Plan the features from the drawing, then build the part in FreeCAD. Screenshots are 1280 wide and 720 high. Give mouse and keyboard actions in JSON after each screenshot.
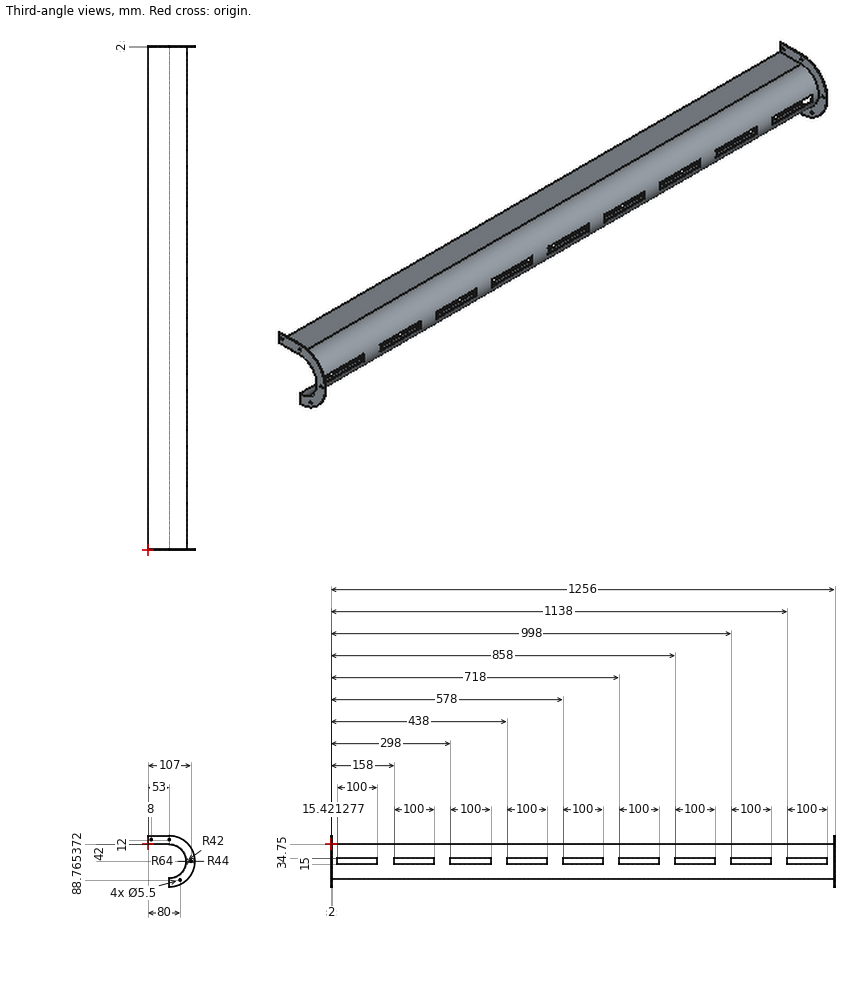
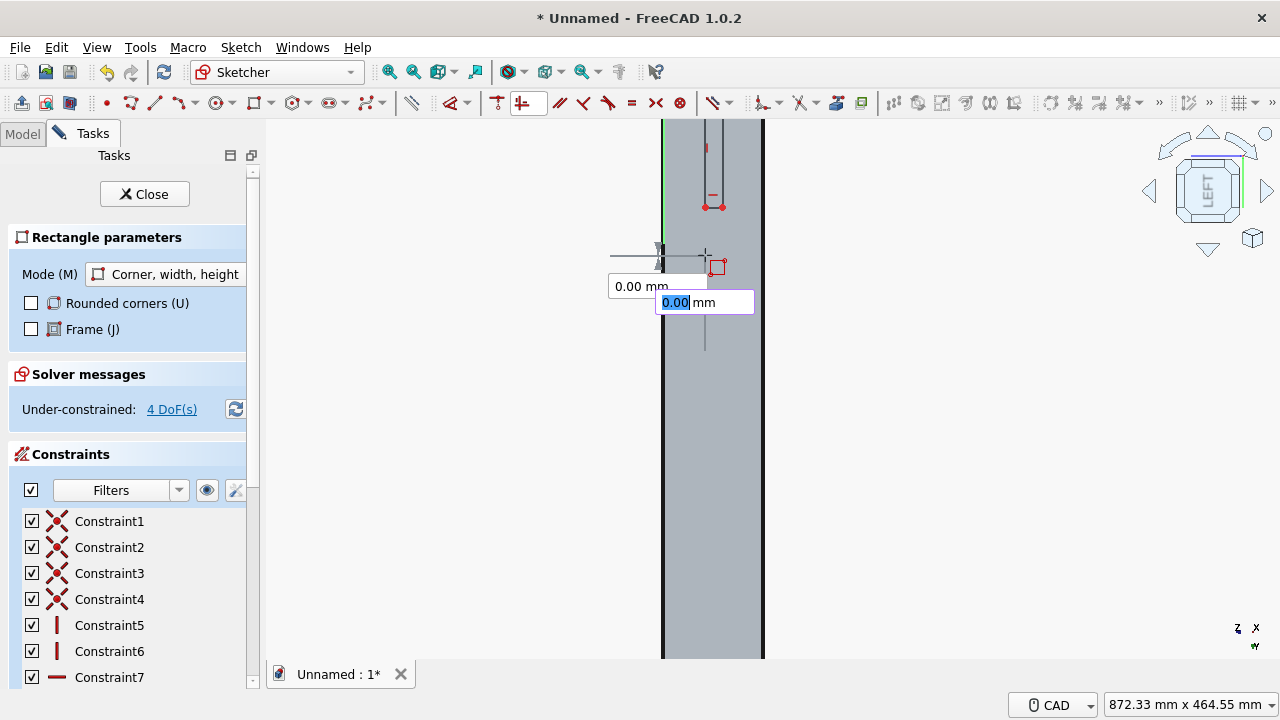
{"action": "scroll", "coordinate": [708, 258], "scroll_direction": "down", "scroll_amount": 7}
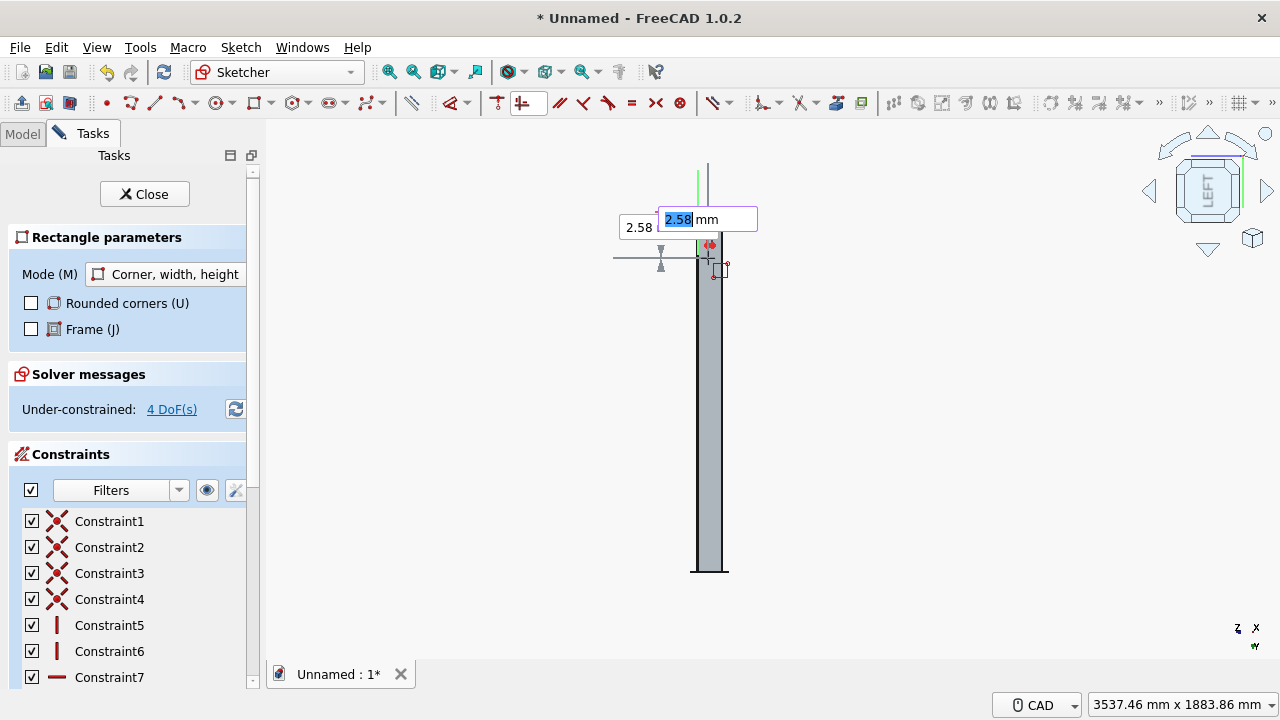
{"action": "left_click", "coordinate": [712, 286]}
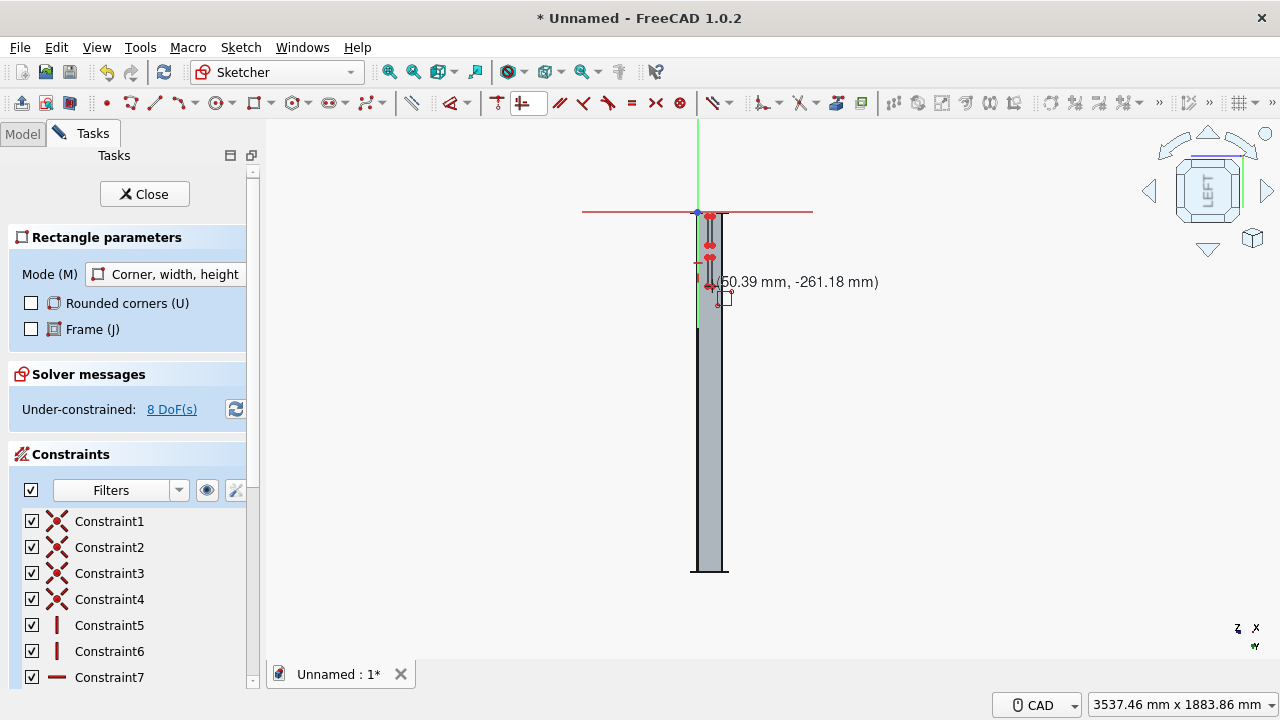
{"action": "scroll", "coordinate": [708, 498], "scroll_direction": "up", "scroll_amount": 7}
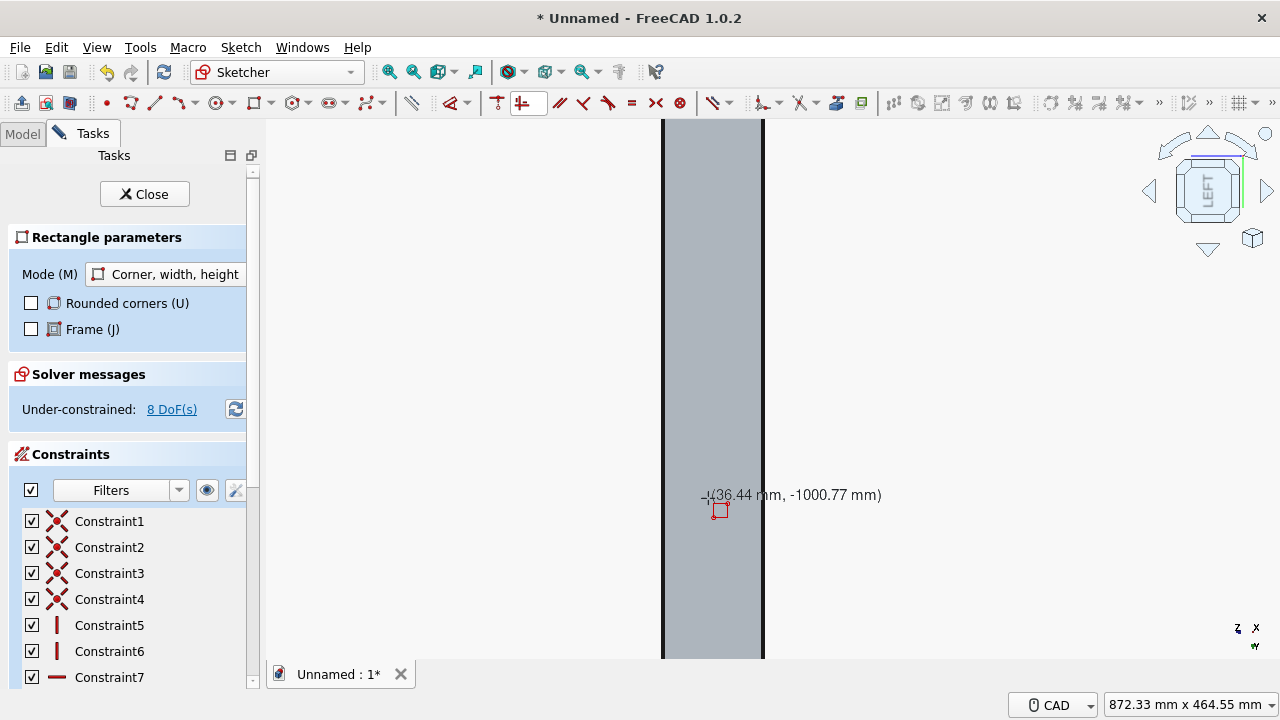
{"action": "left_click", "coordinate": [705, 497]}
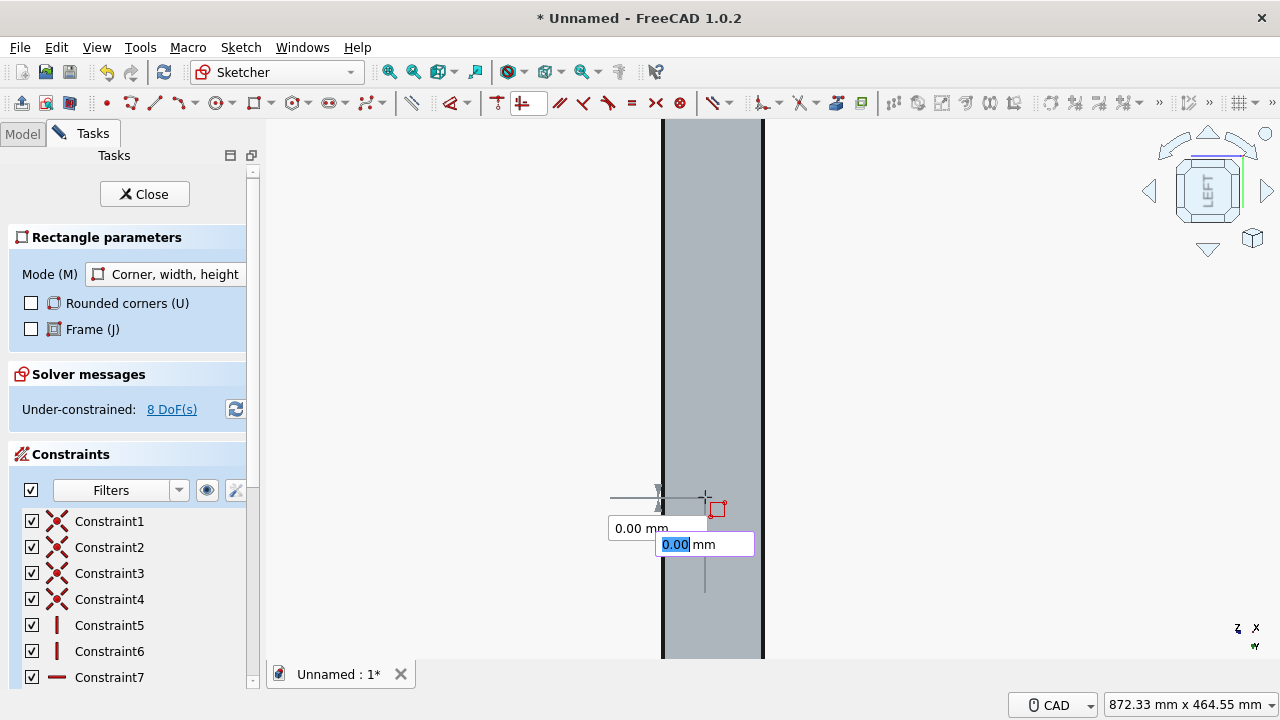
{"action": "scroll", "coordinate": [708, 498], "scroll_direction": "down", "scroll_amount": 7}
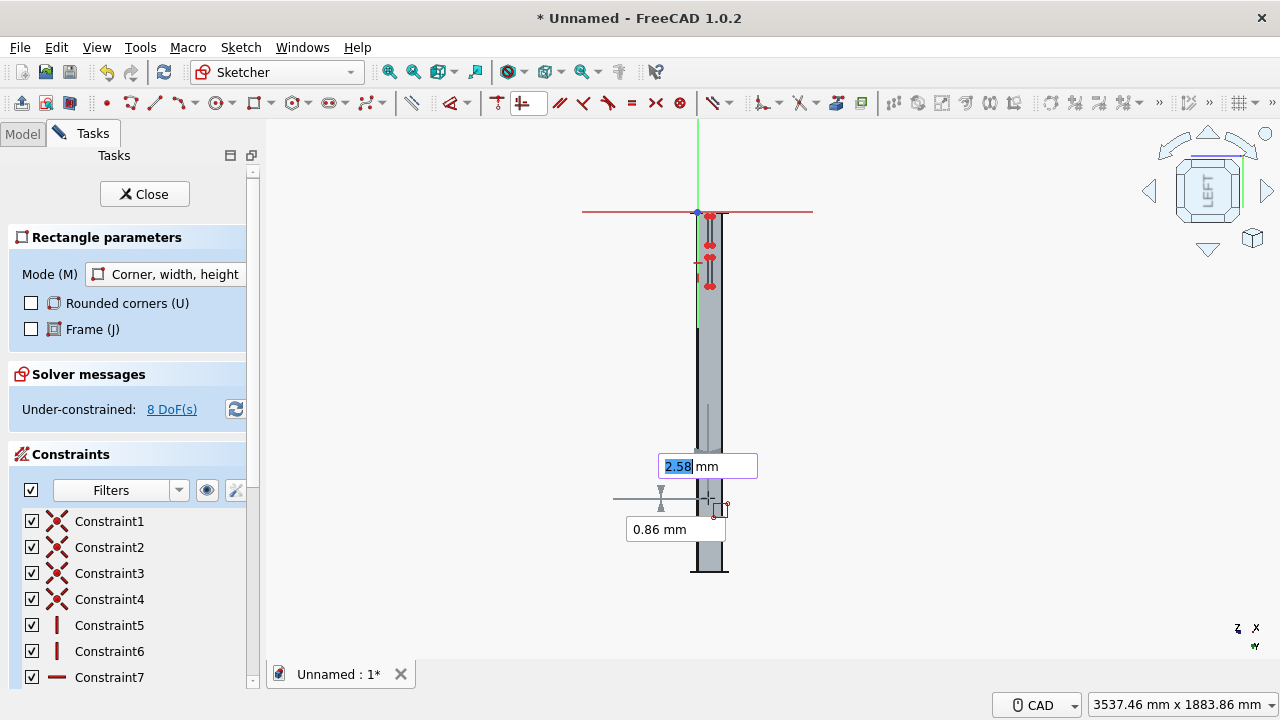
{"action": "left_click", "coordinate": [712, 527]}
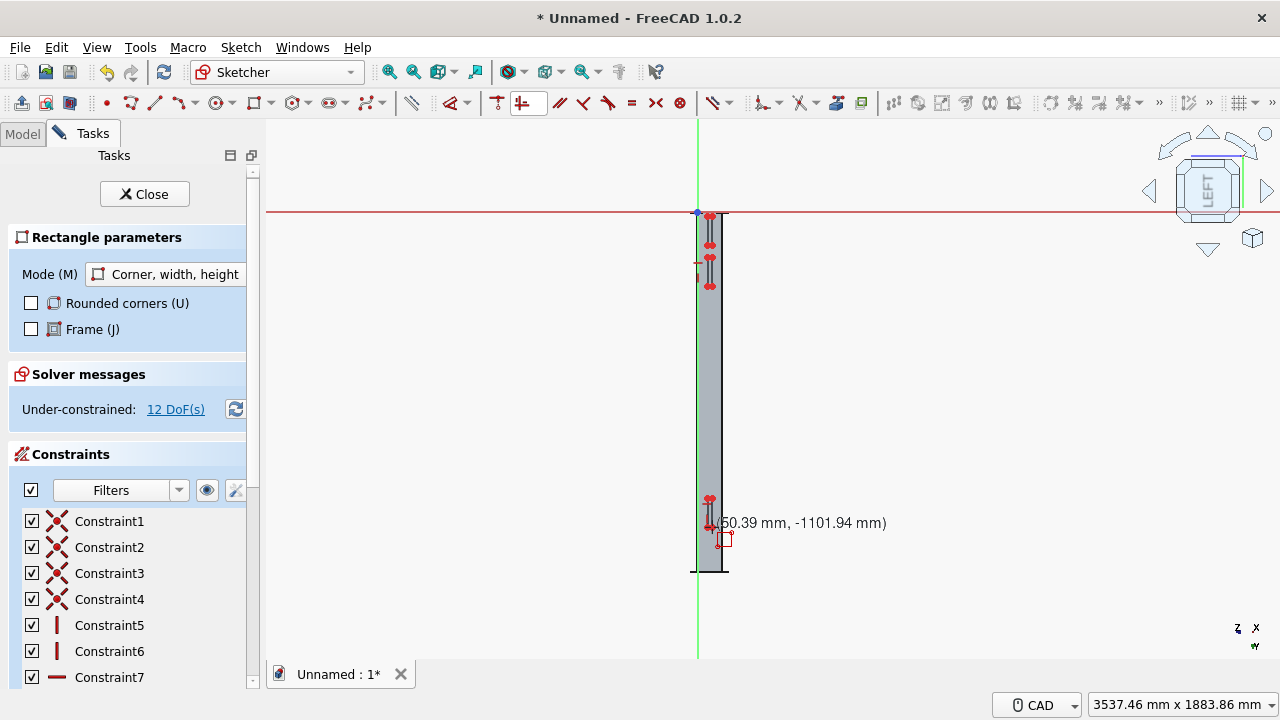
{"action": "scroll", "coordinate": [708, 298], "scroll_direction": "up", "scroll_amount": 7}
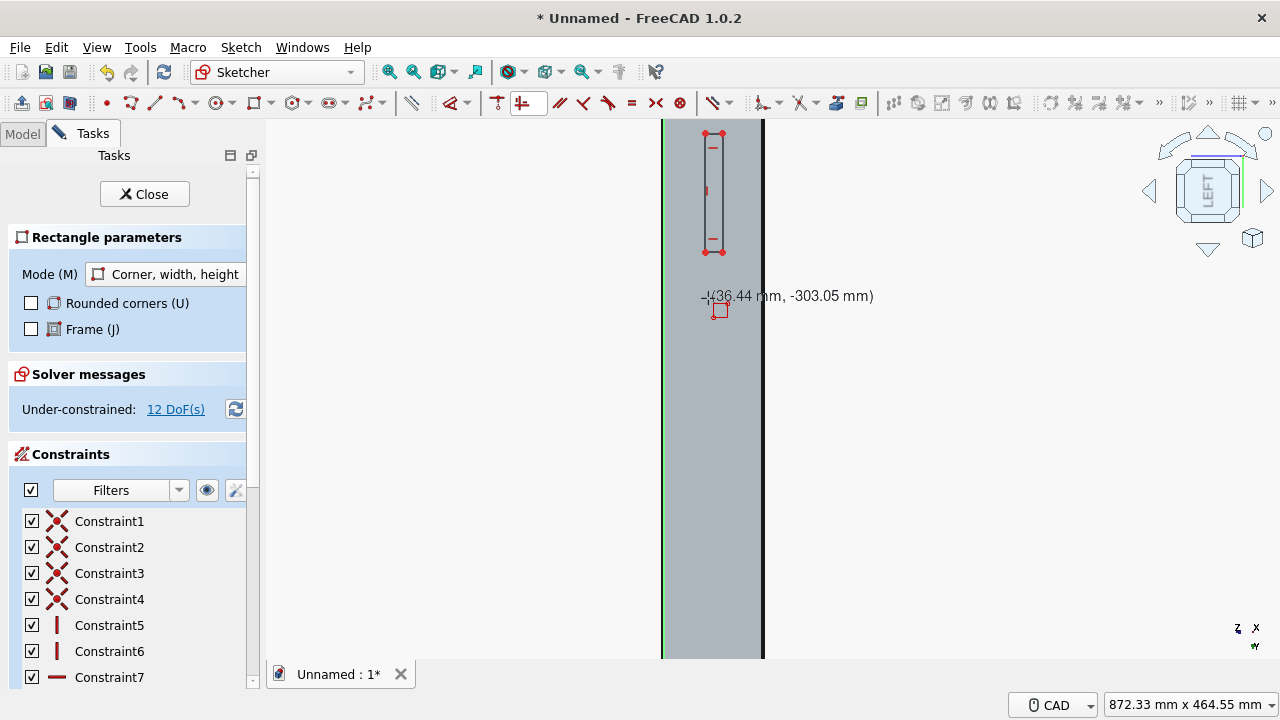
{"action": "left_click", "coordinate": [705, 295]}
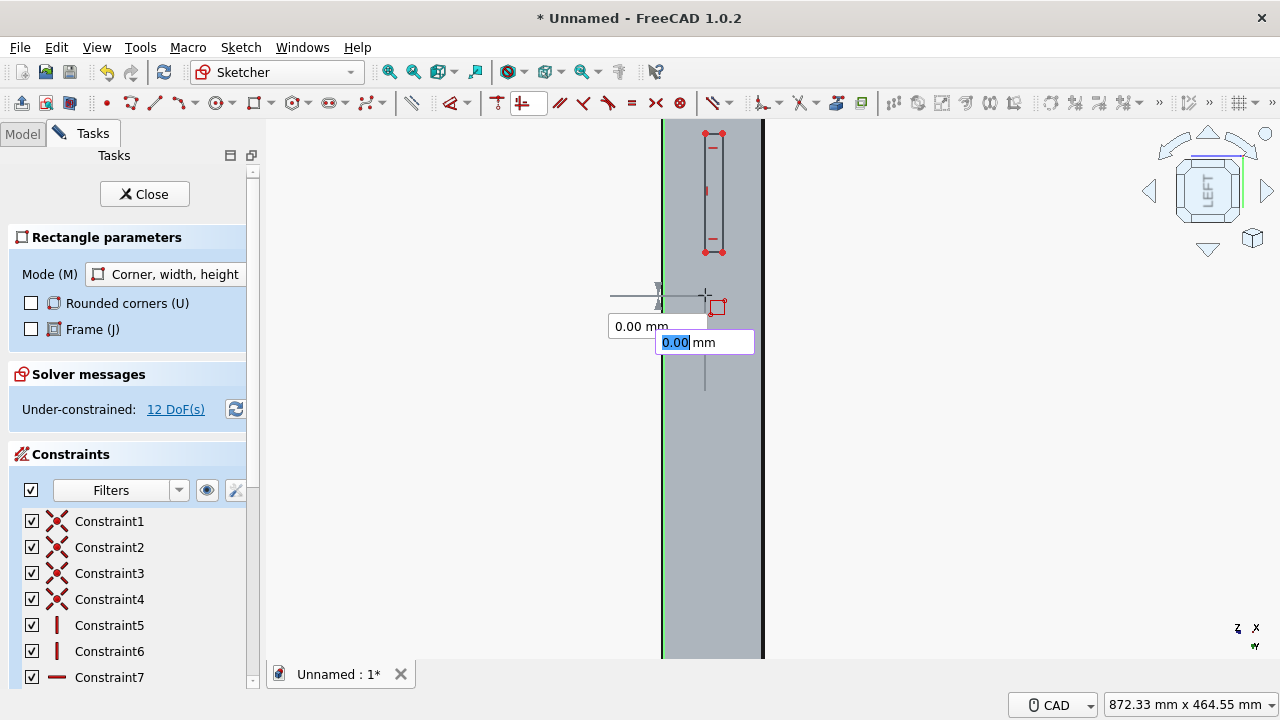
{"action": "scroll", "coordinate": [708, 298], "scroll_direction": "down", "scroll_amount": 7}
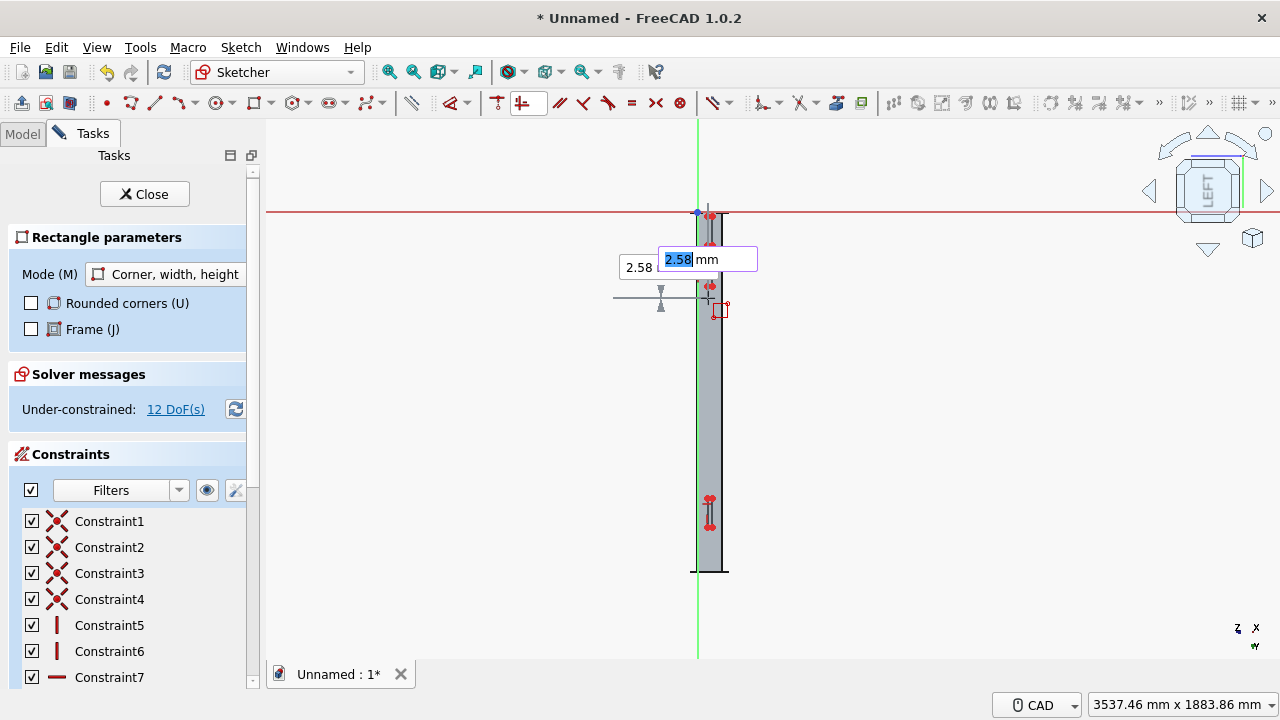
{"action": "left_click", "coordinate": [712, 326]}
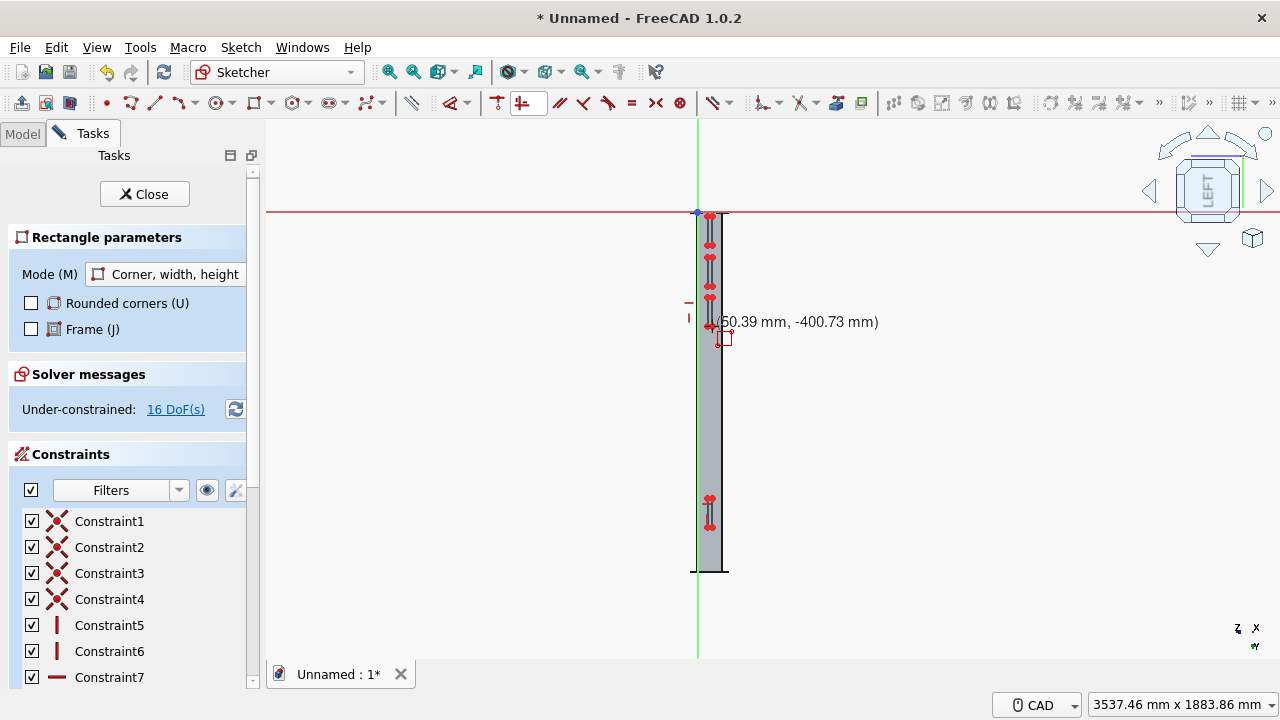
{"action": "scroll", "coordinate": [708, 338], "scroll_direction": "up", "scroll_amount": 7}